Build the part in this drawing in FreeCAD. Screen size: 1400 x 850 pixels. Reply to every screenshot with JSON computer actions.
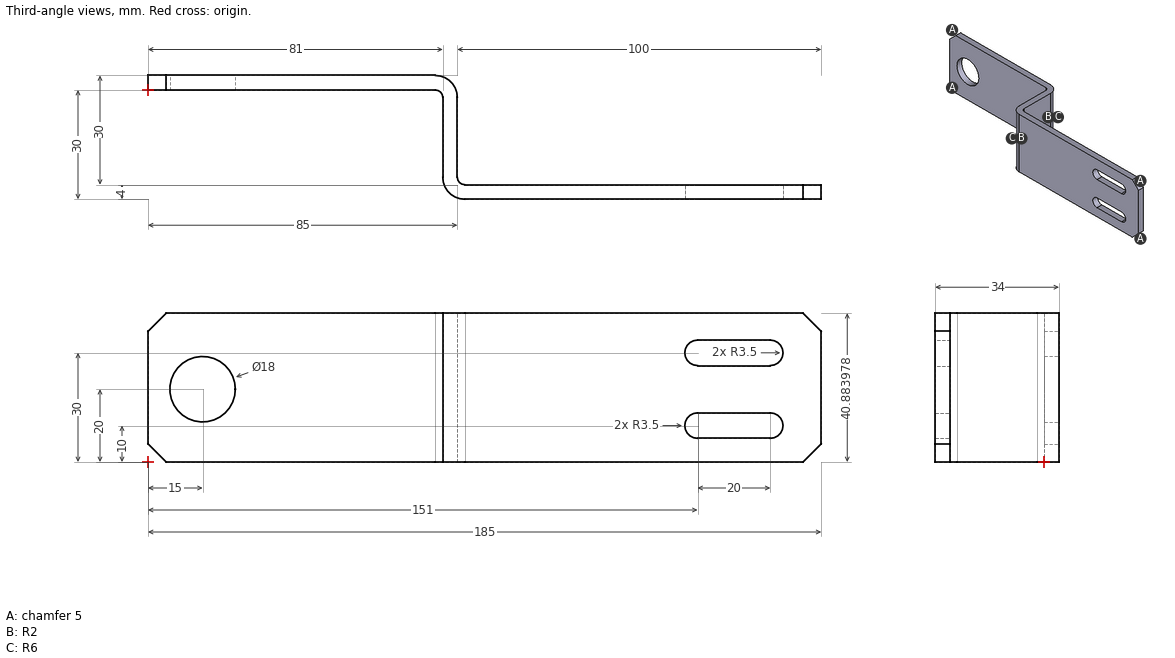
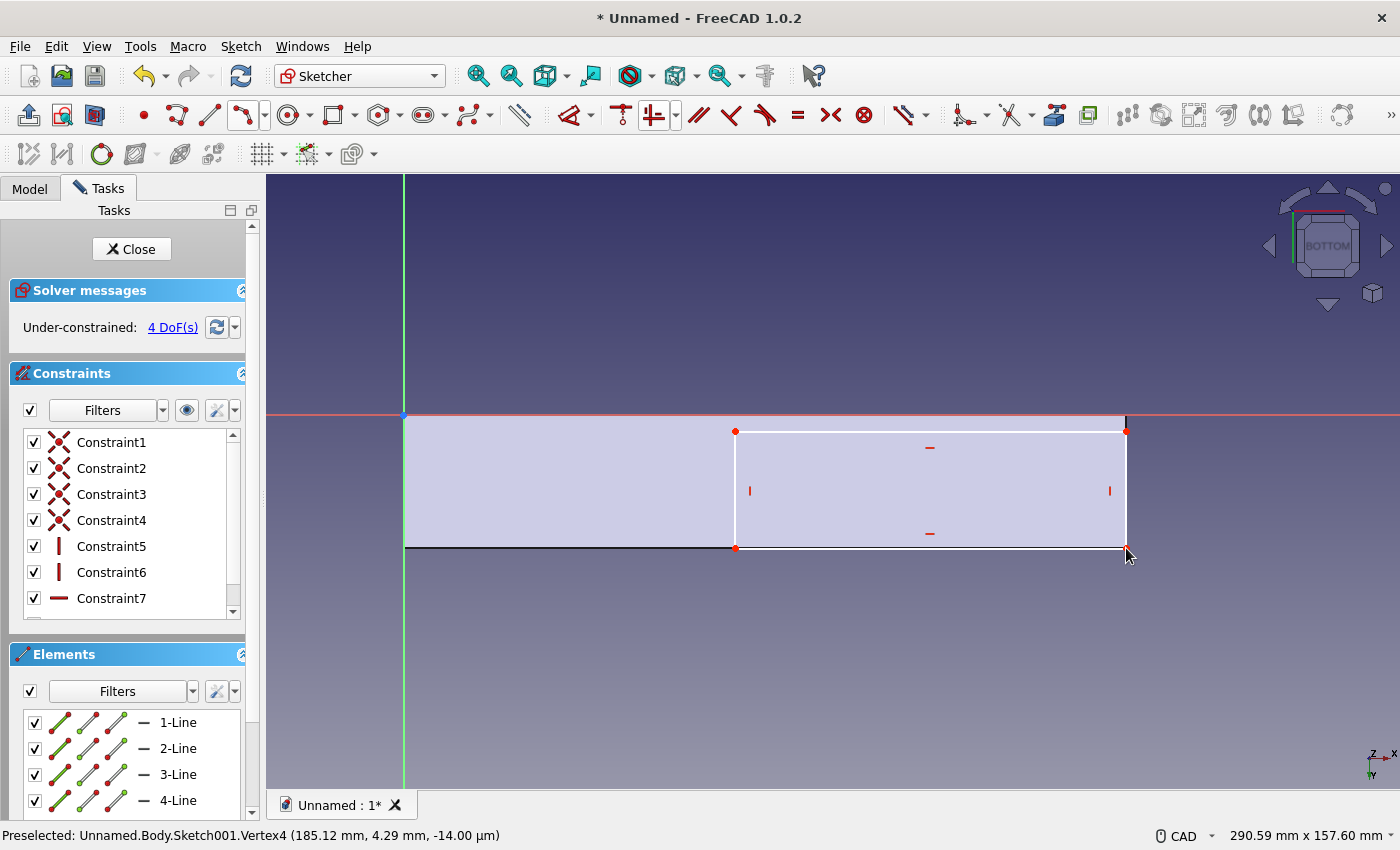
{"action": "left_click", "coordinate": [568, 116]}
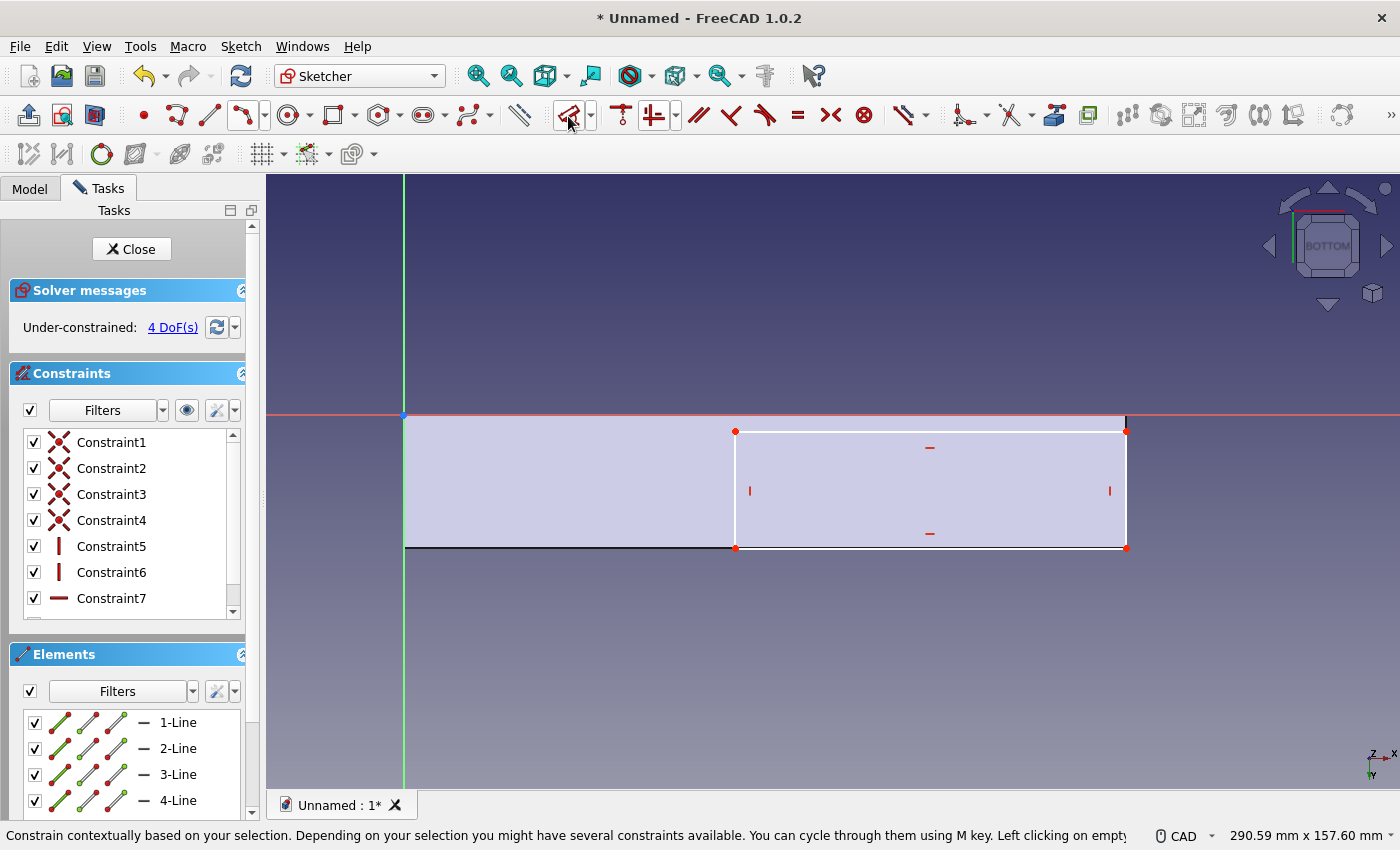
{"action": "left_click", "coordinate": [735, 467]}
{"action": "left_click", "coordinate": [701, 490]}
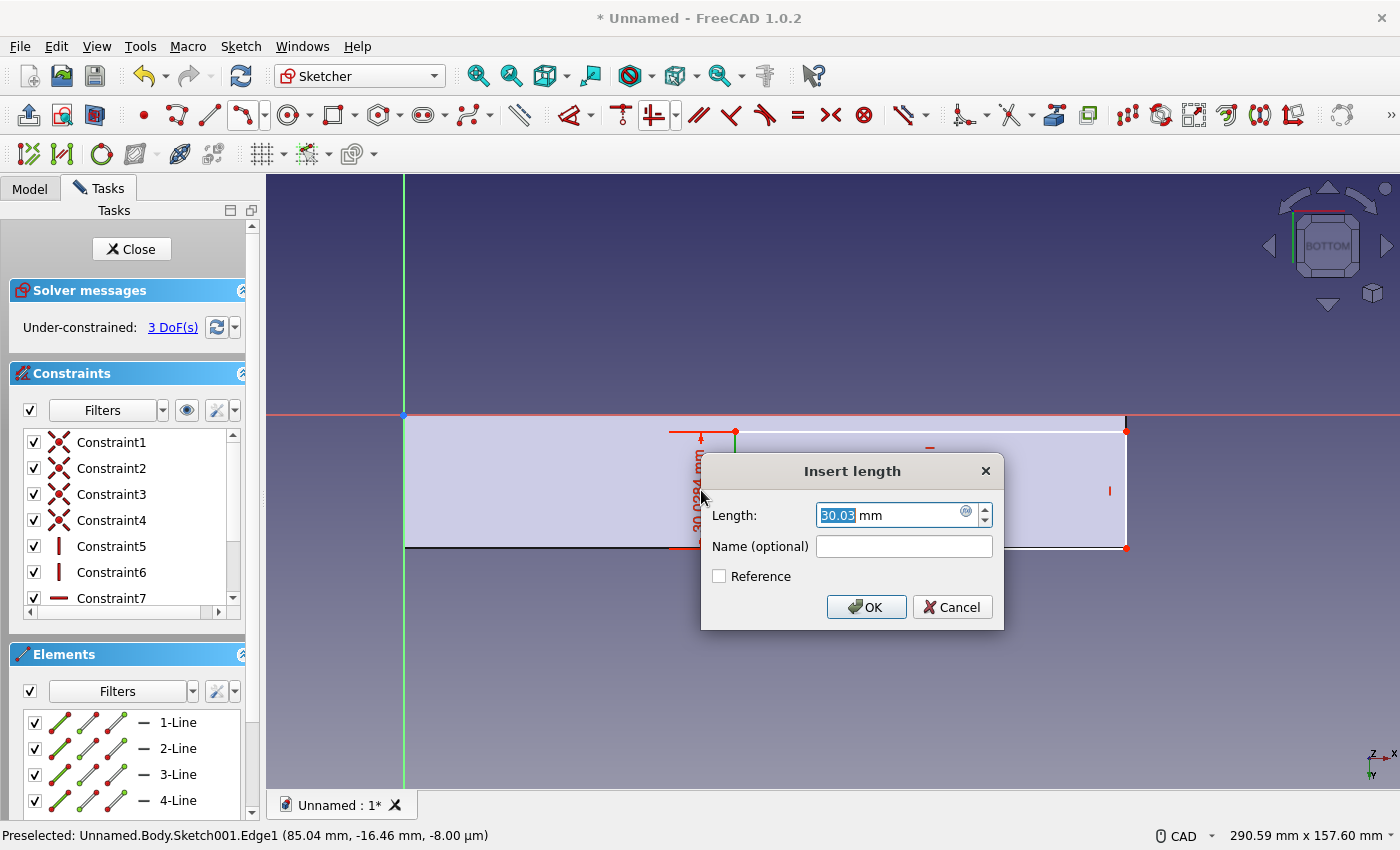
{"action": "type", "text": "30"}
{"action": "key", "text": "Return"}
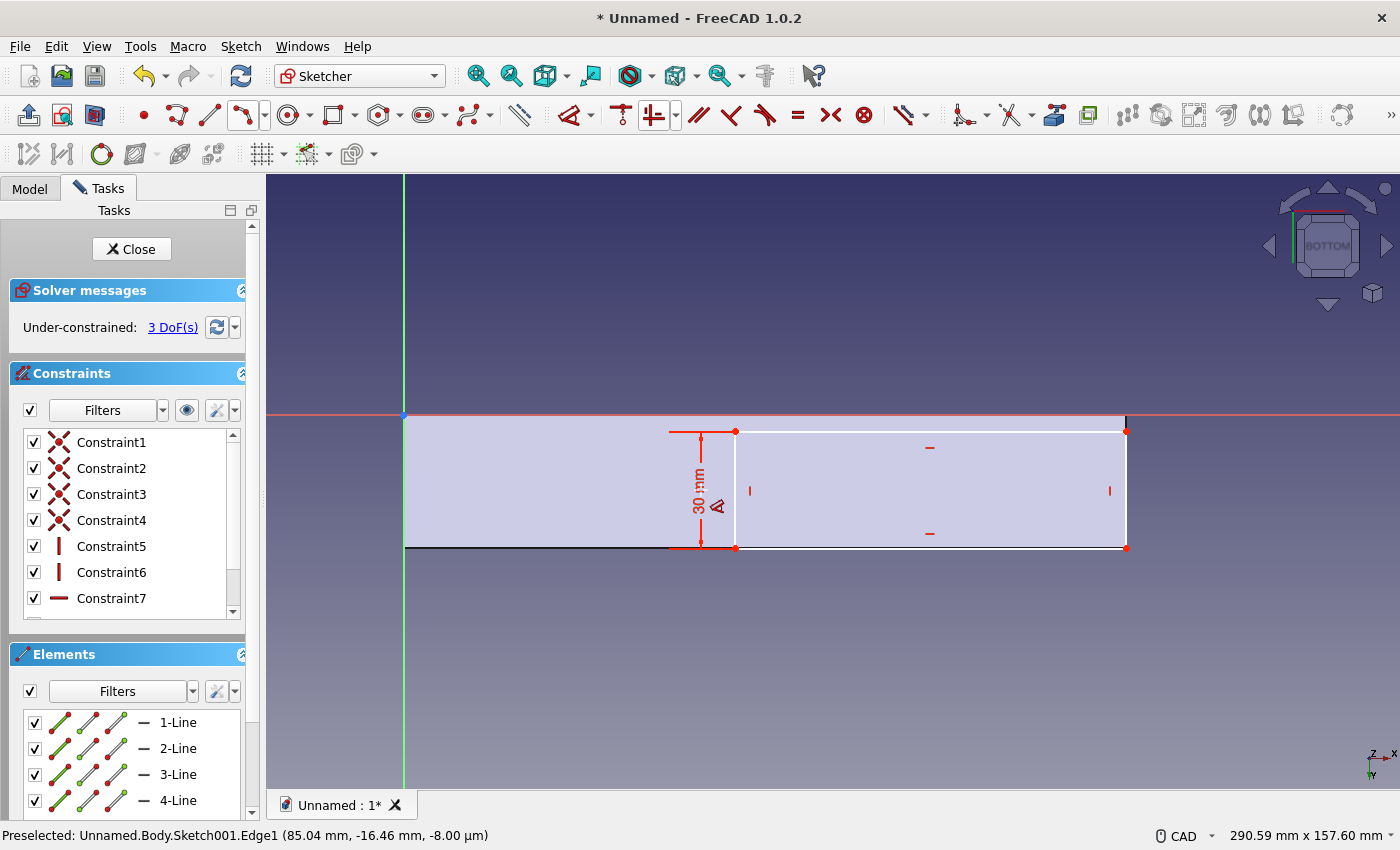
{"action": "scroll", "coordinate": [735, 432], "scroll_direction": "up", "scroll_amount": 5}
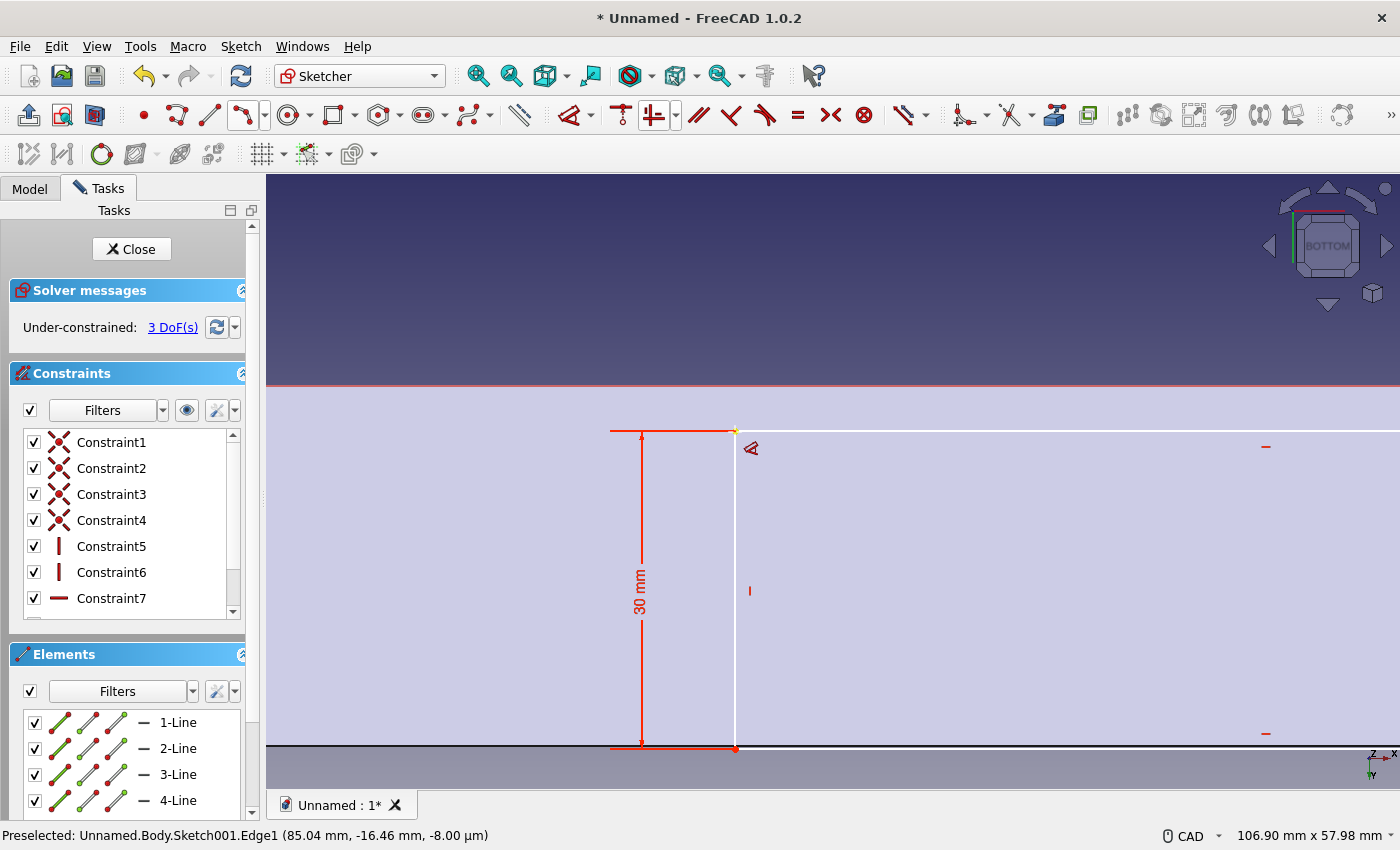
{"action": "left_click", "coordinate": [735, 431]}
{"action": "left_click", "coordinate": [769, 408]}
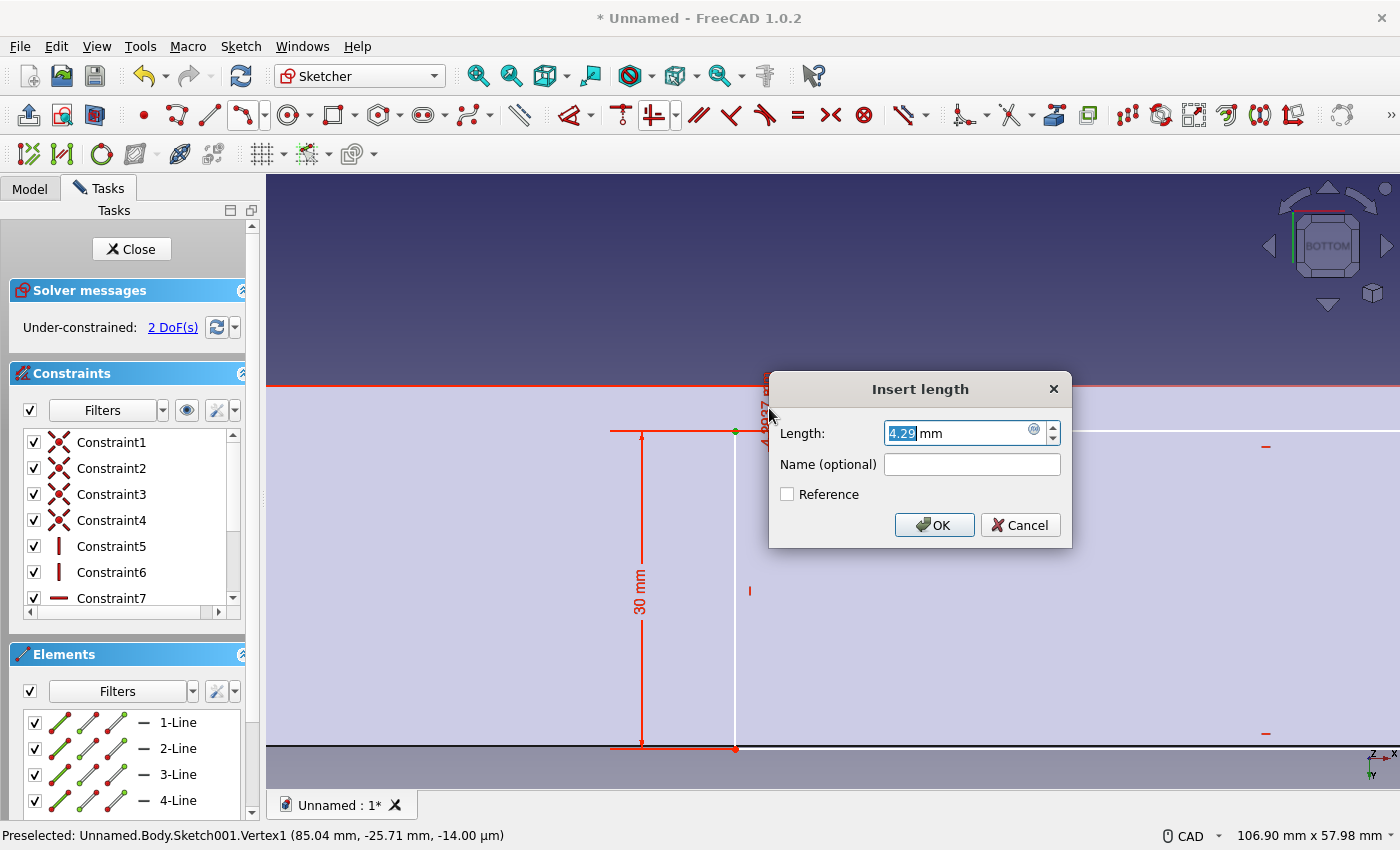
{"action": "type", "text": "4"}
{"action": "key", "text": "Return"}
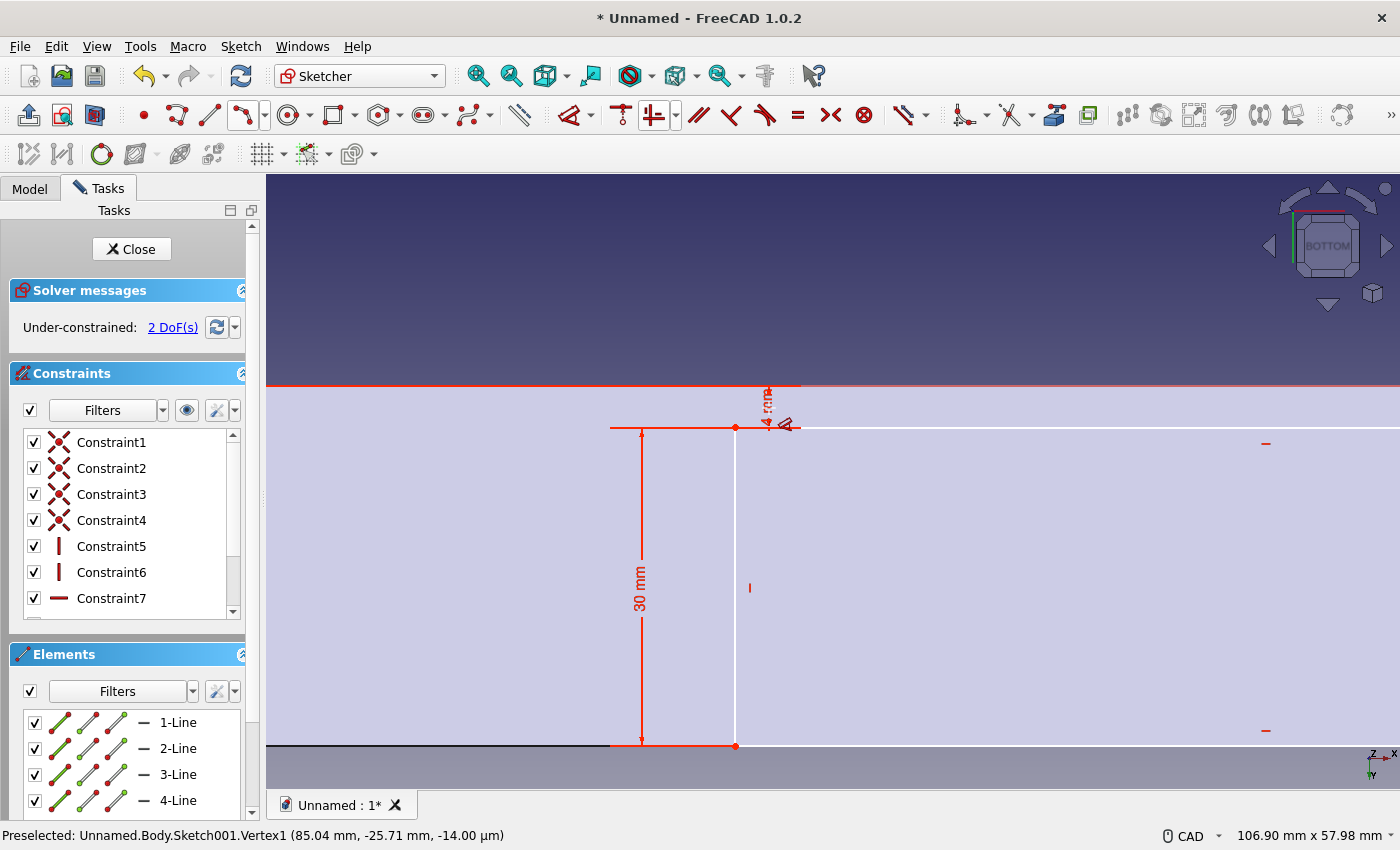
{"action": "left_click", "coordinate": [1054, 746]}
{"action": "left_click", "coordinate": [985, 712]}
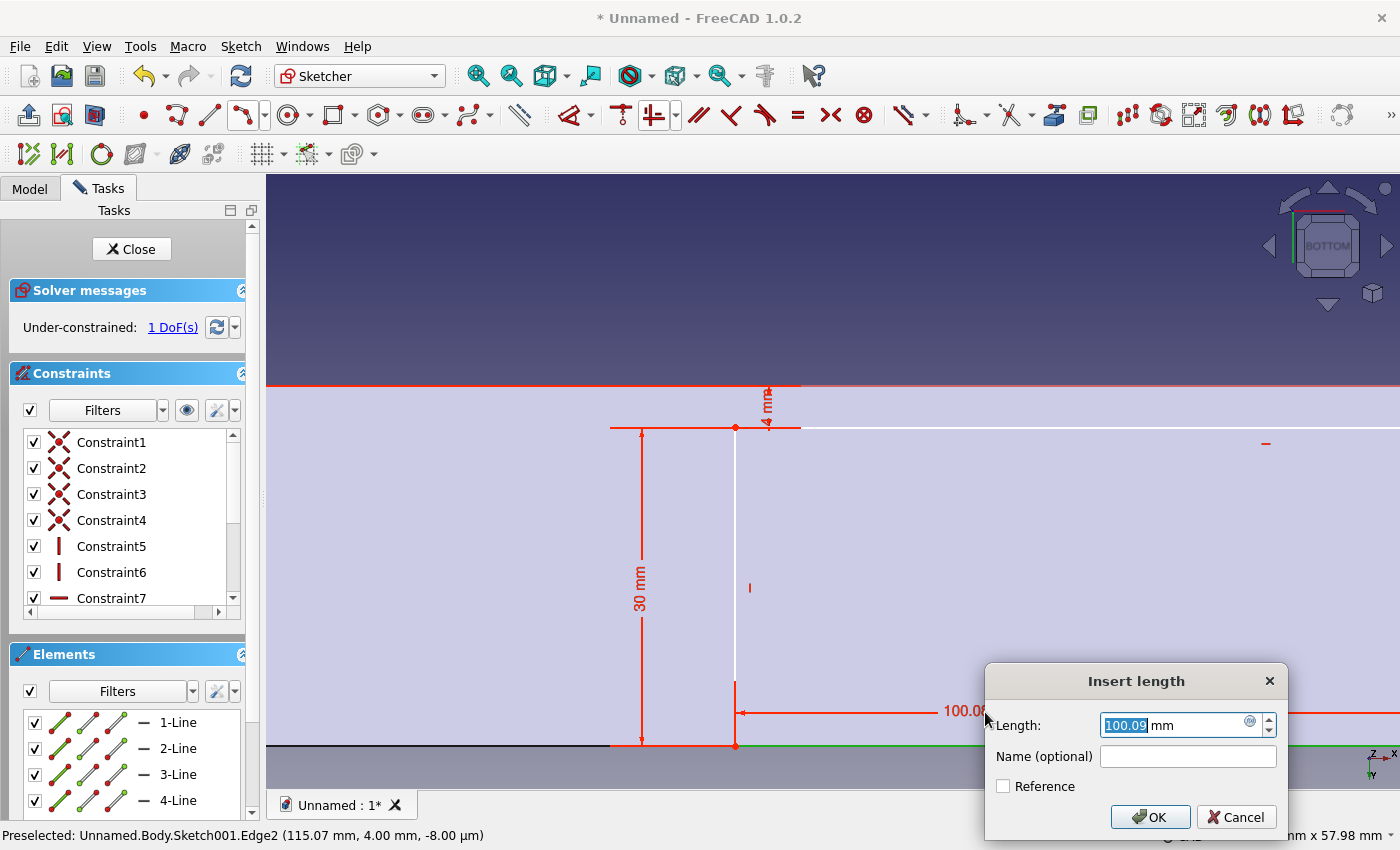
{"action": "type", "text": "100"}
{"action": "key", "text": "Return"}